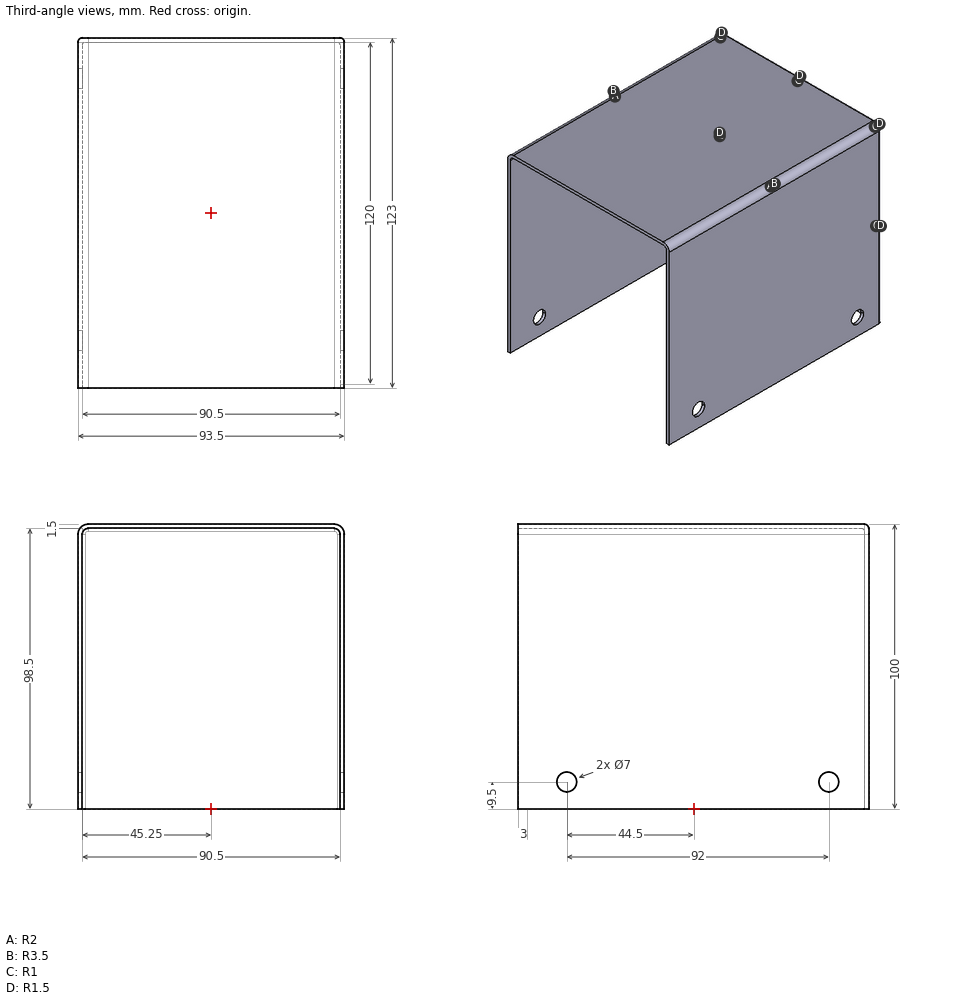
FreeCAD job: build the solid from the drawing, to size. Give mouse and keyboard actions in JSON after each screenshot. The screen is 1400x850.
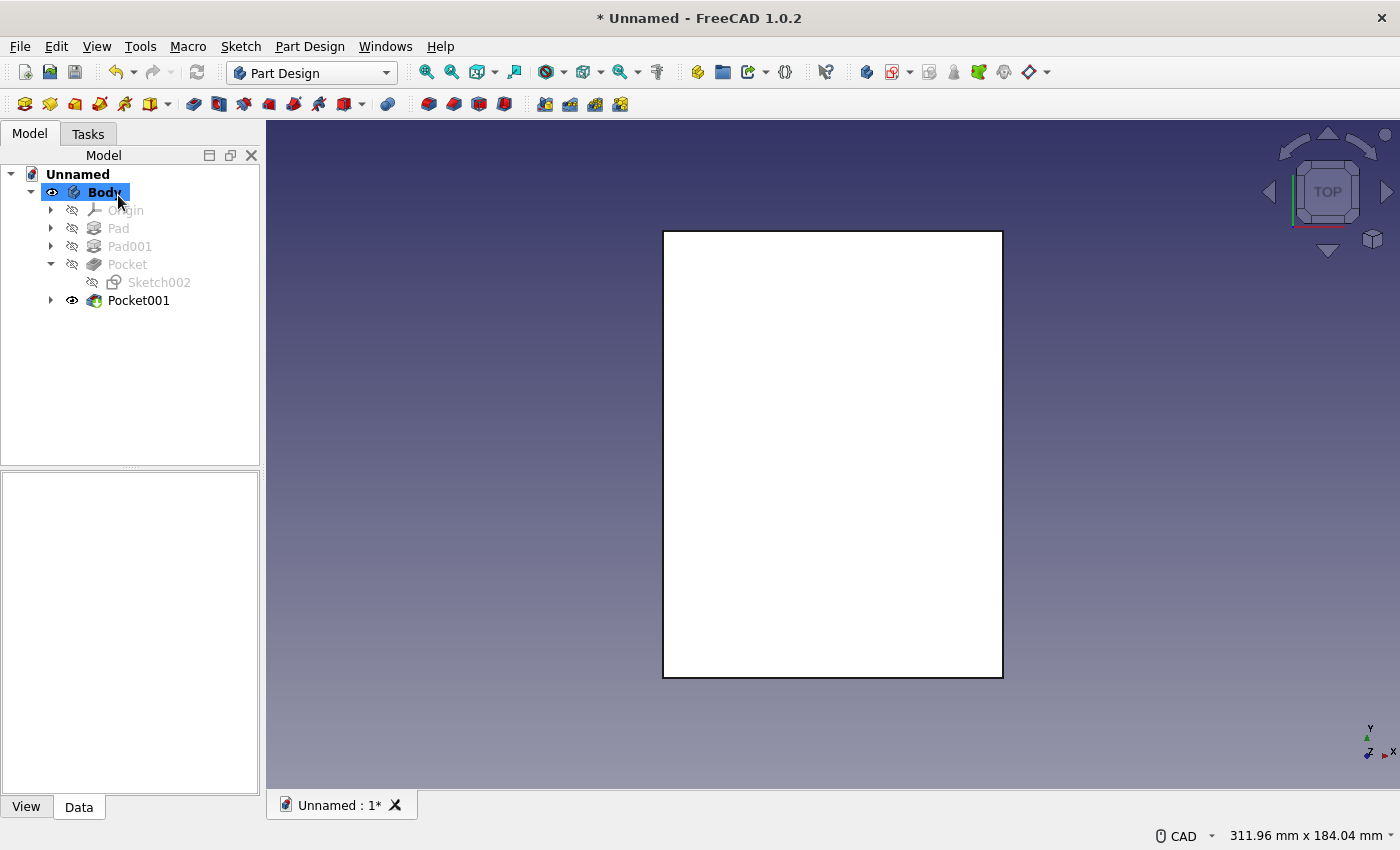
{"action": "key", "text": "1"}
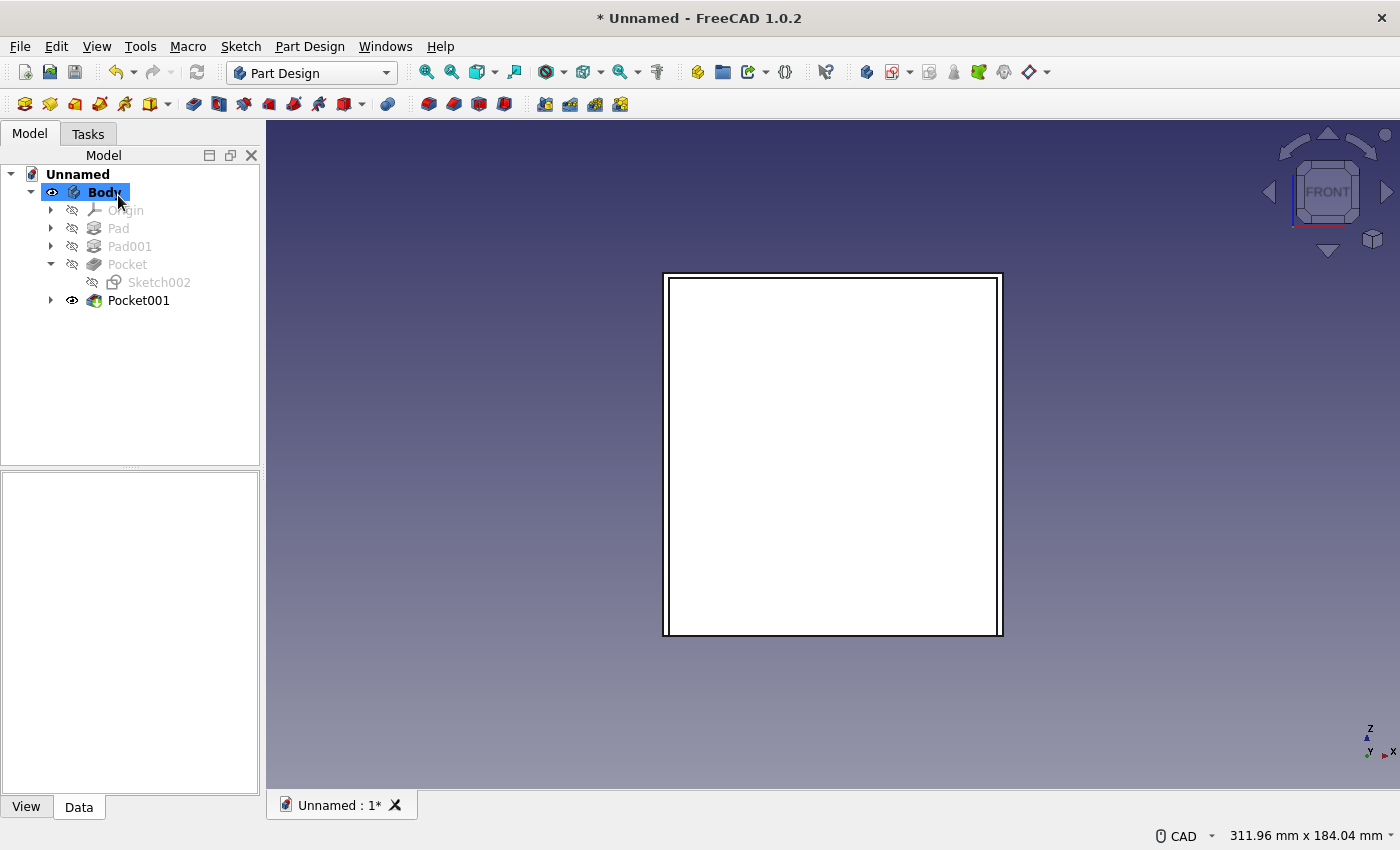
{"action": "key", "text": "3"}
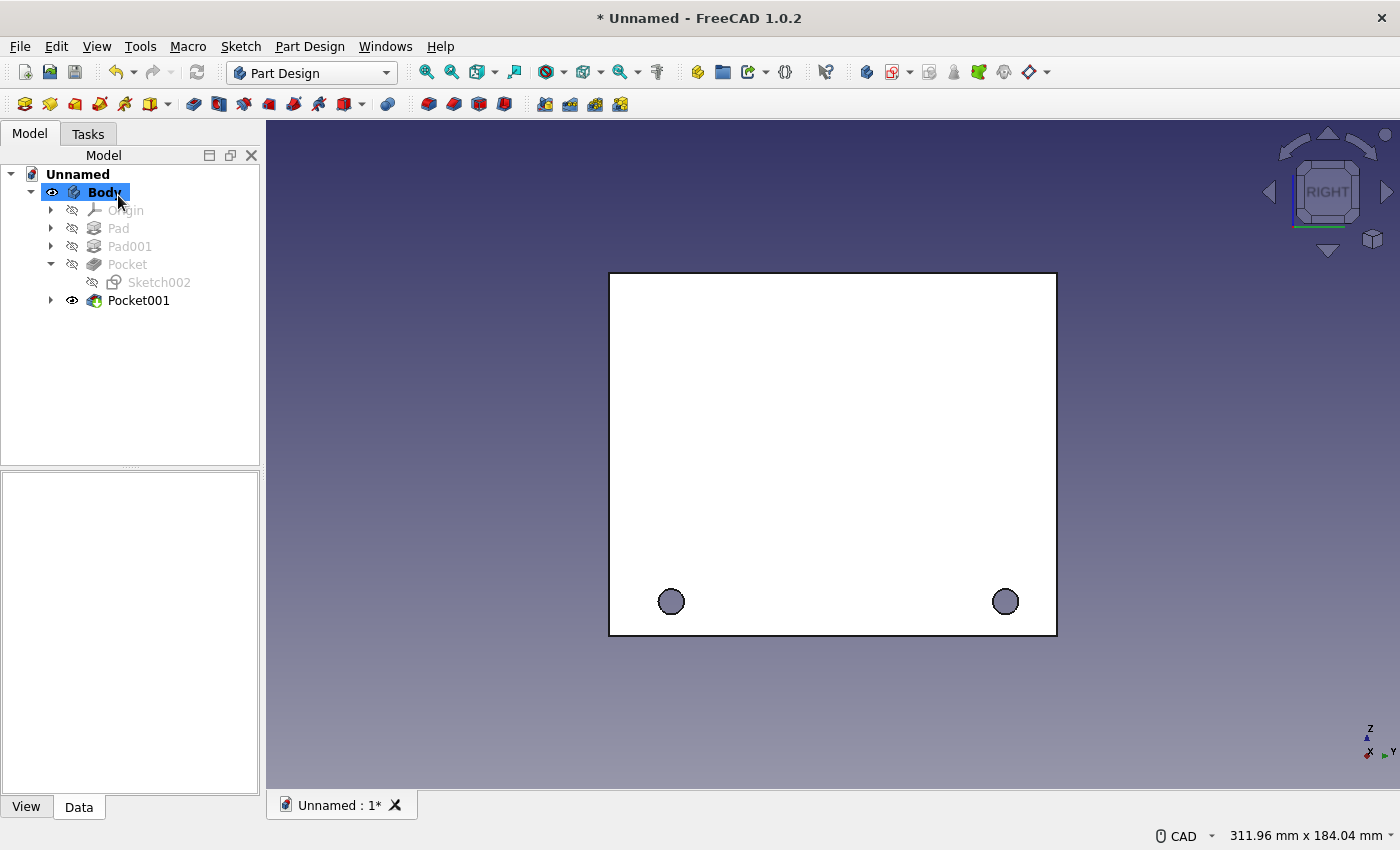
{"action": "key", "text": "5"}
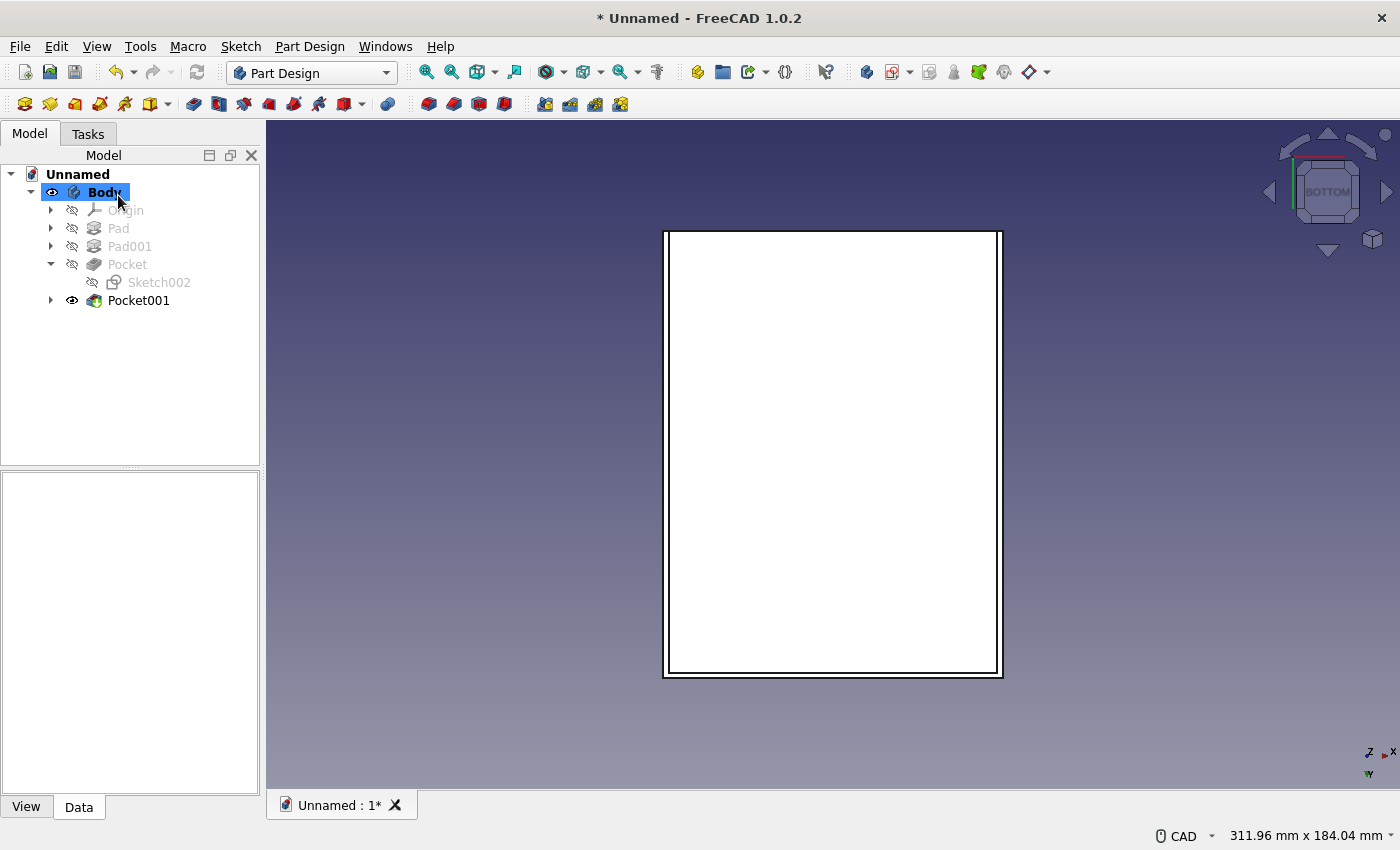
{"action": "key", "text": "4"}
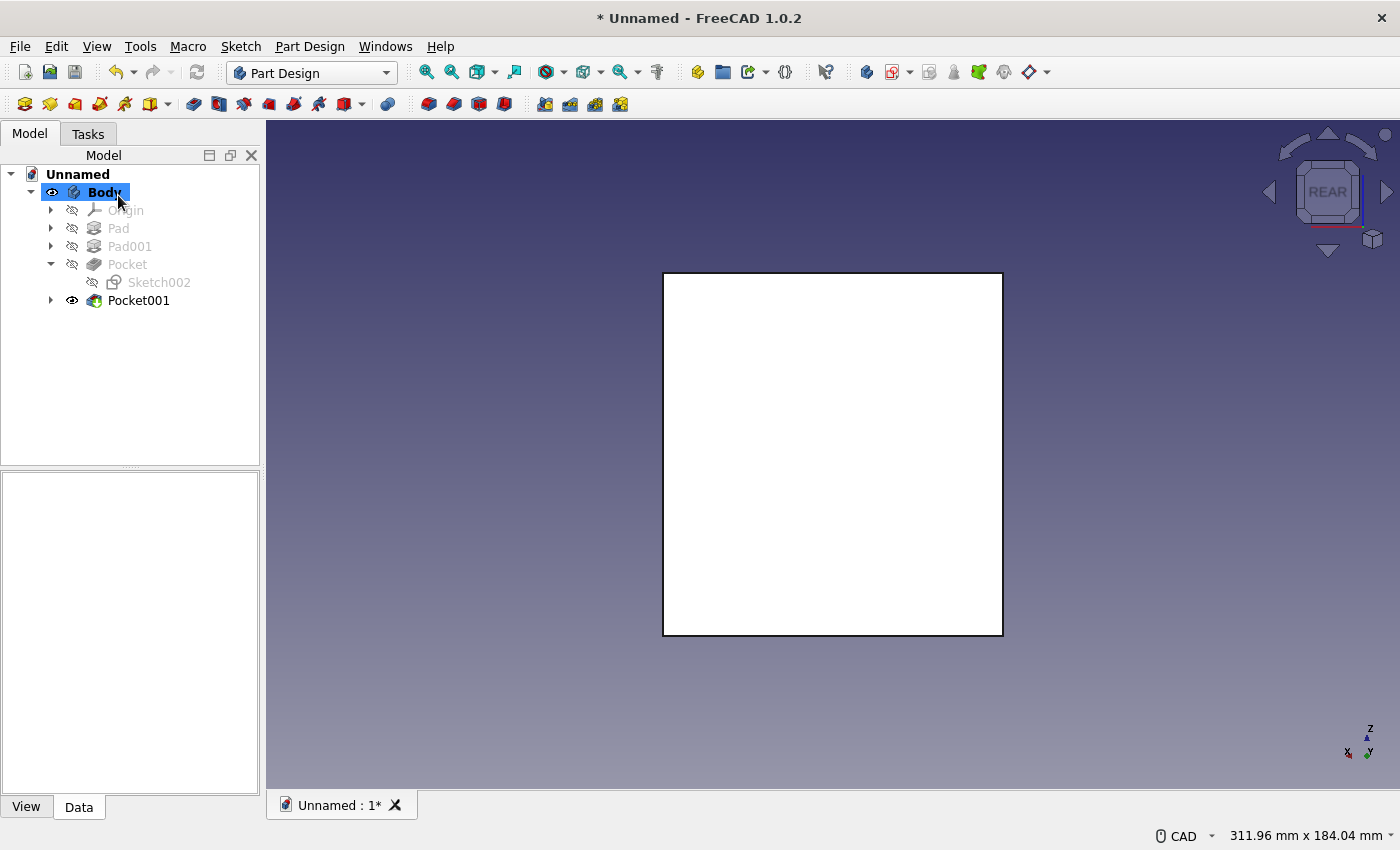
{"action": "key", "text": "6"}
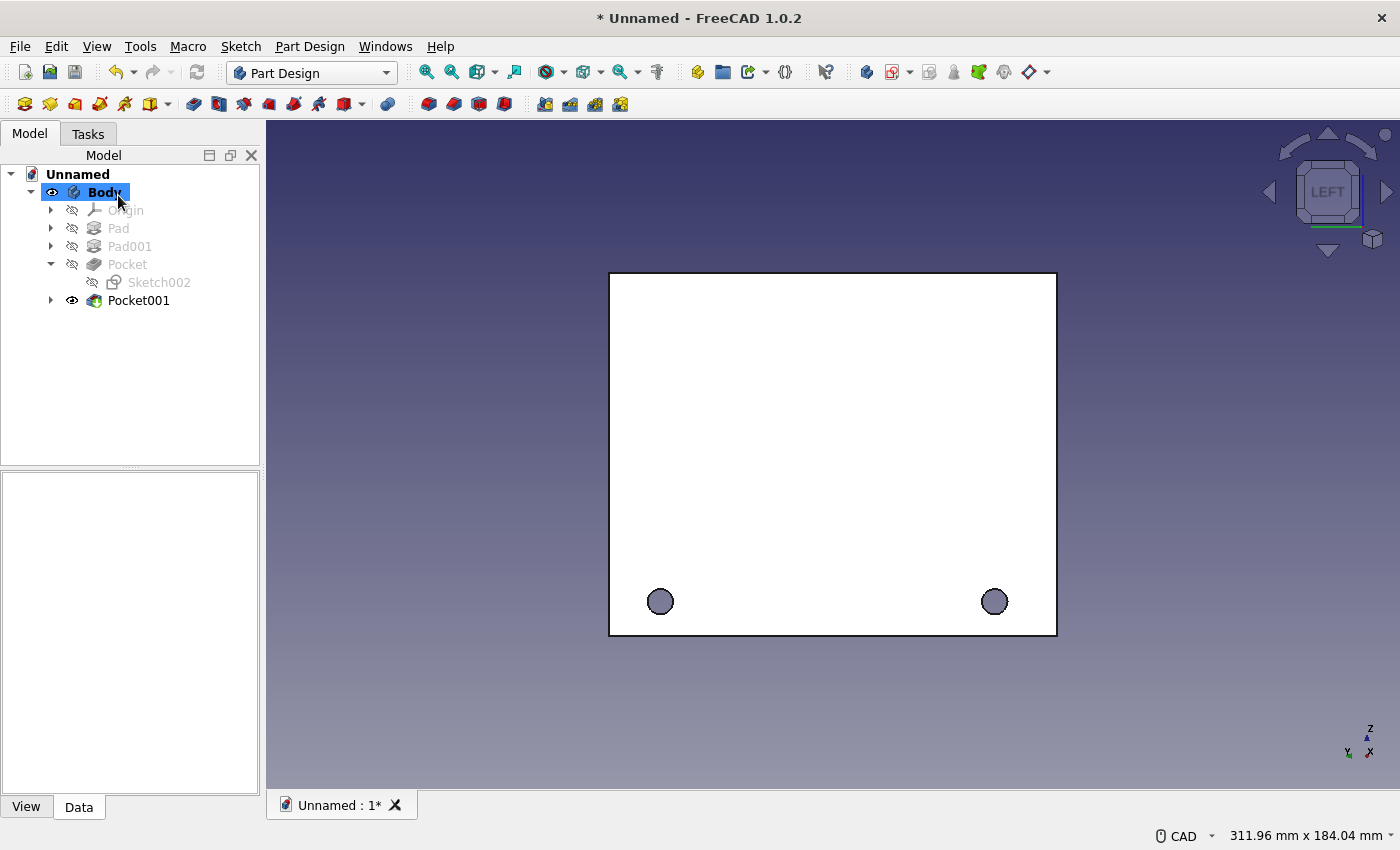
{"action": "key", "text": "v 3"}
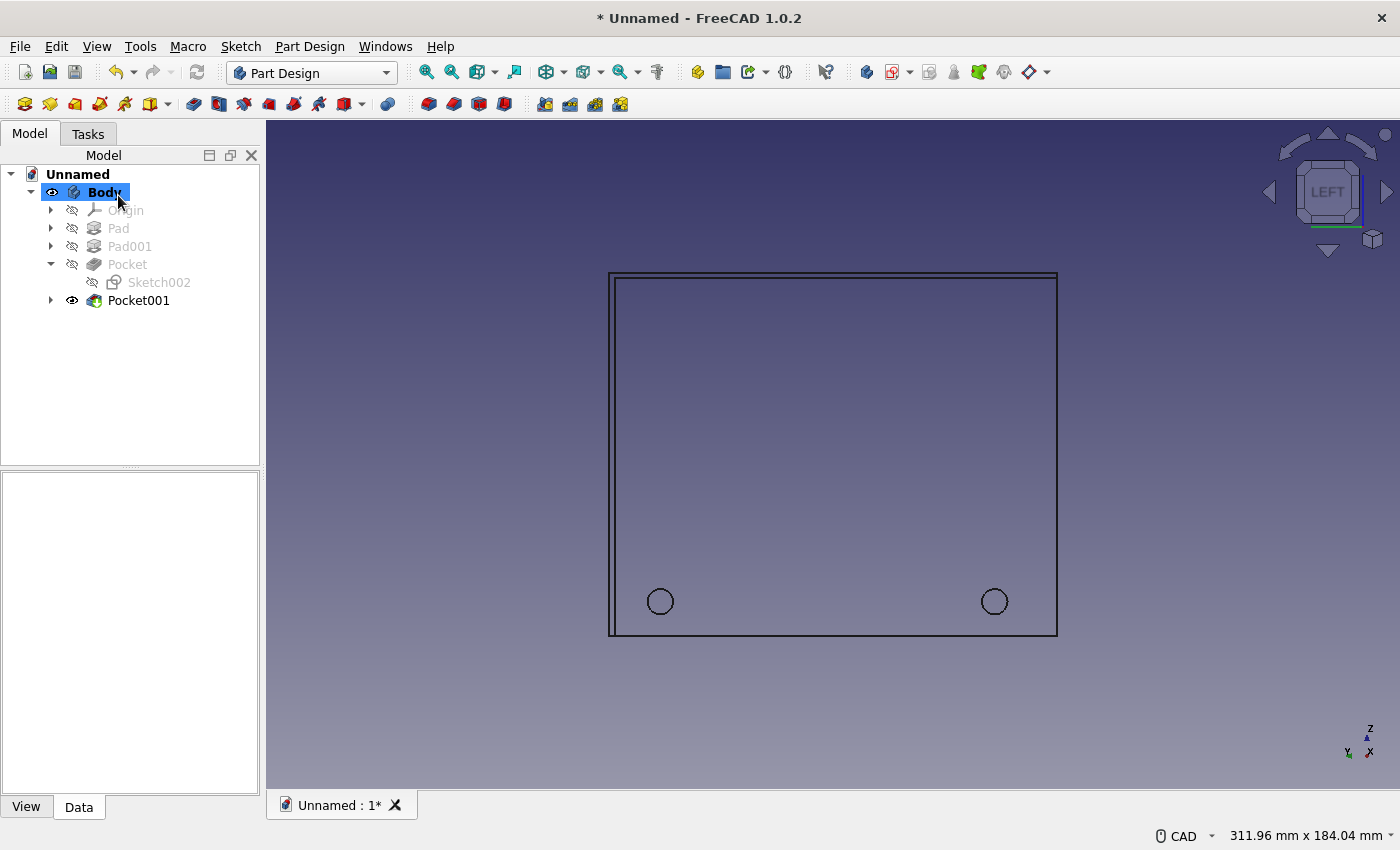
{"action": "key", "text": "0"}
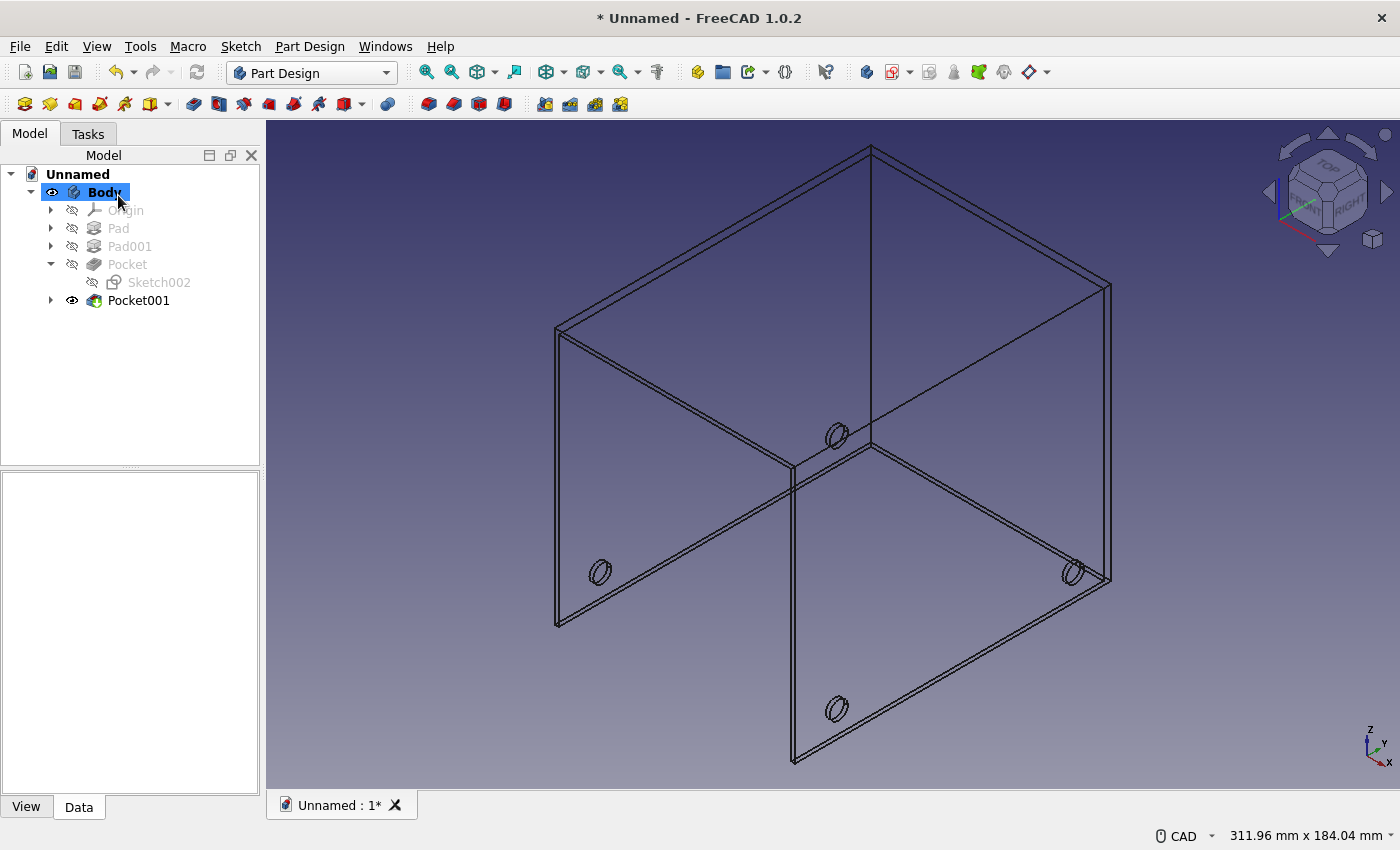
{"action": "left_click", "coordinate": [715, 244]}